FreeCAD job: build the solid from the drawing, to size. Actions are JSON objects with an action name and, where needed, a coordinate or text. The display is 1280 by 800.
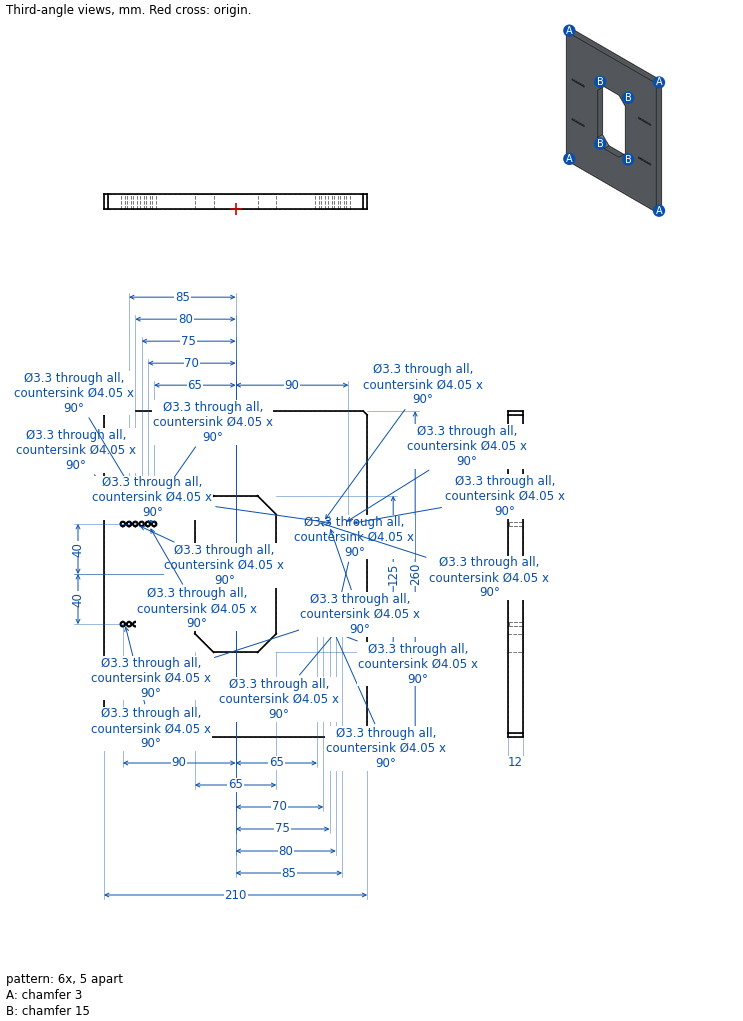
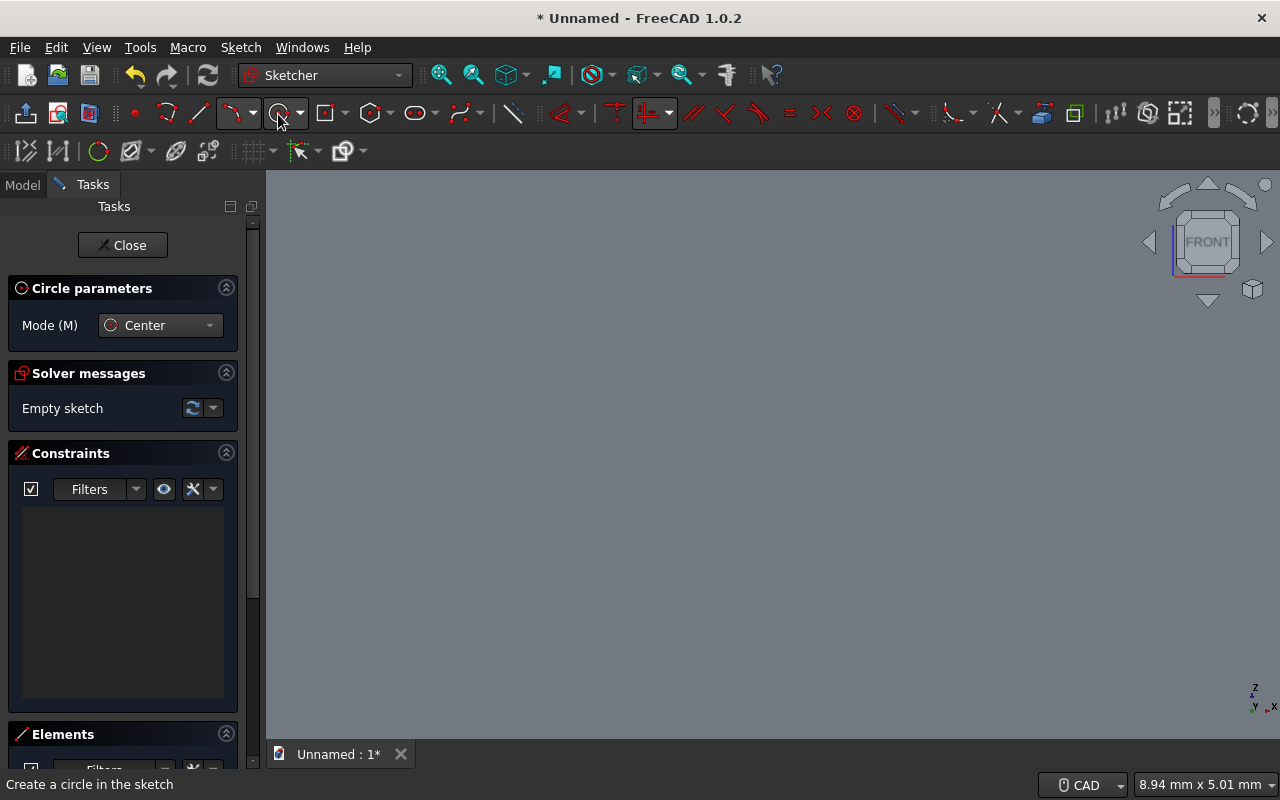
{"action": "left_click", "coordinate": [704, 453]}
{"action": "mouse_move", "coordinate": [836, 320]}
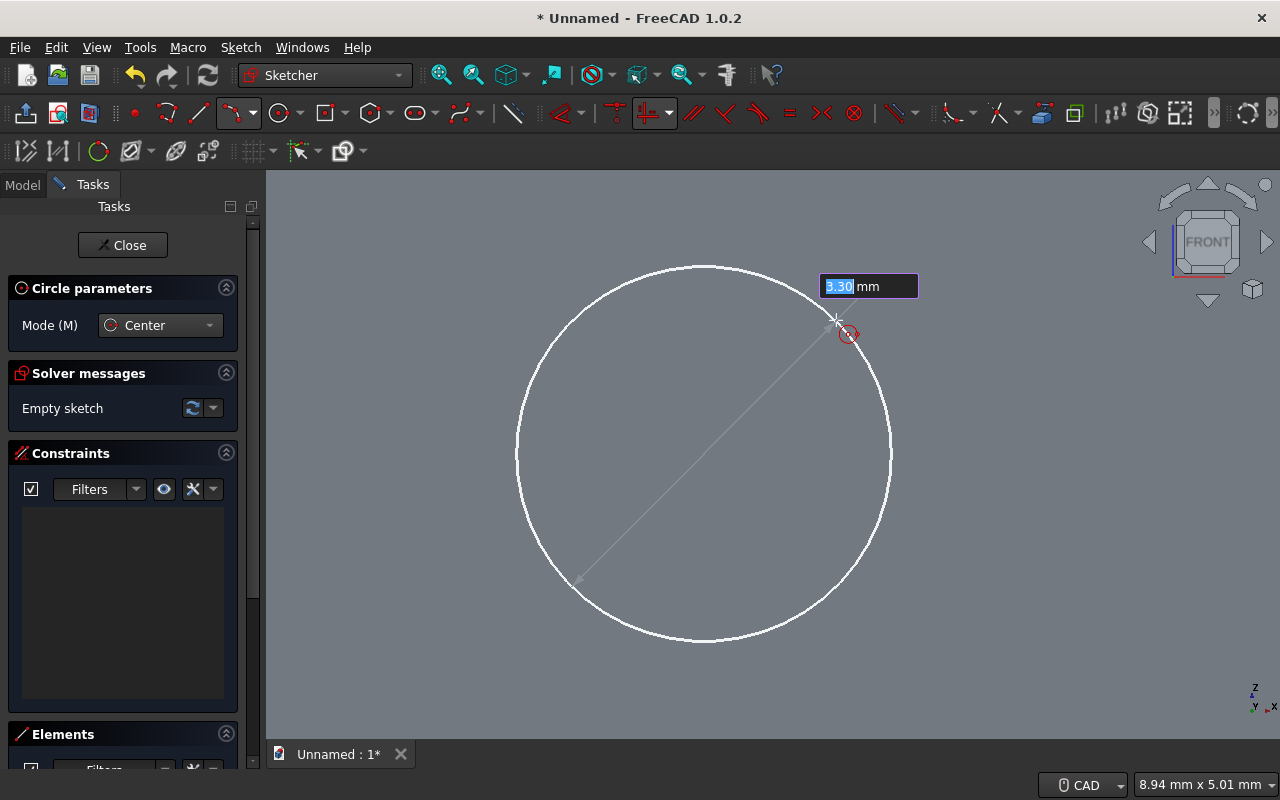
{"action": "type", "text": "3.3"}
{"action": "key", "text": "Return"}
{"action": "key", "text": "Escape"}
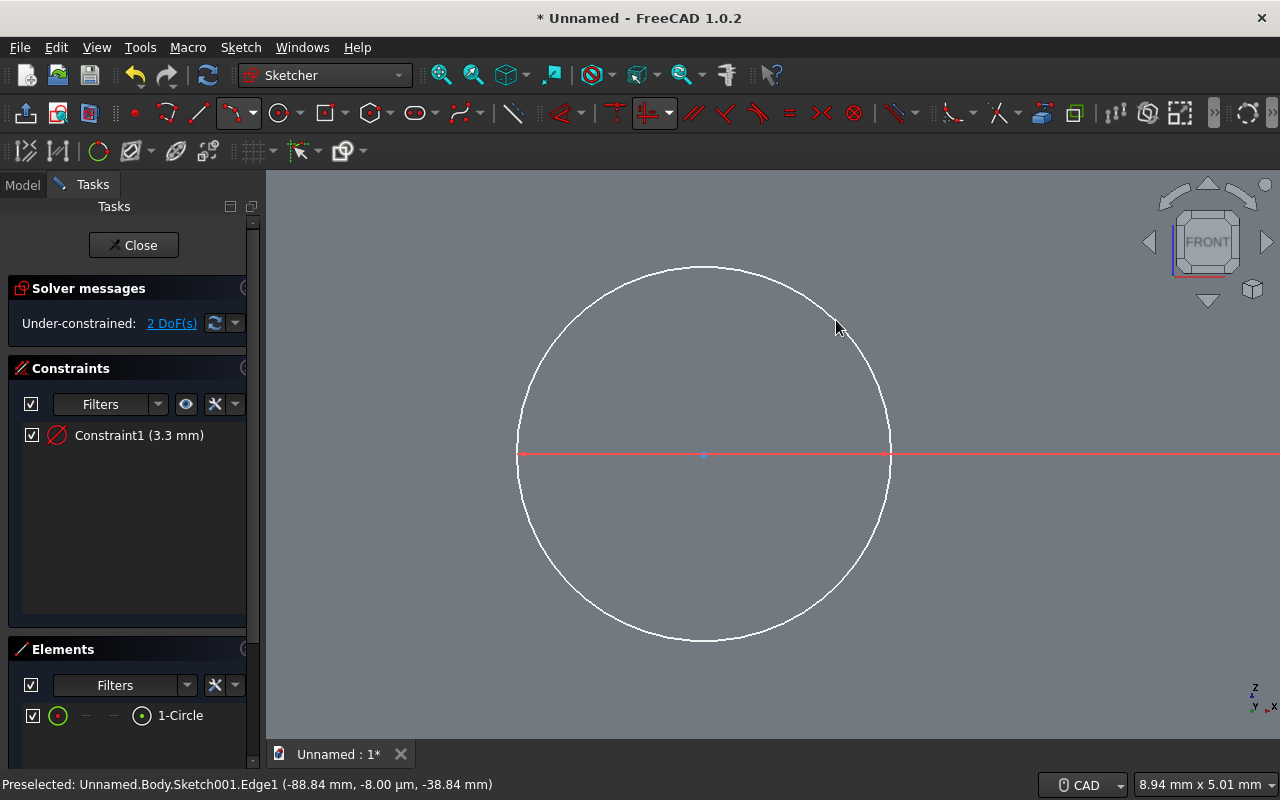
{"action": "left_click", "coordinate": [704, 454]}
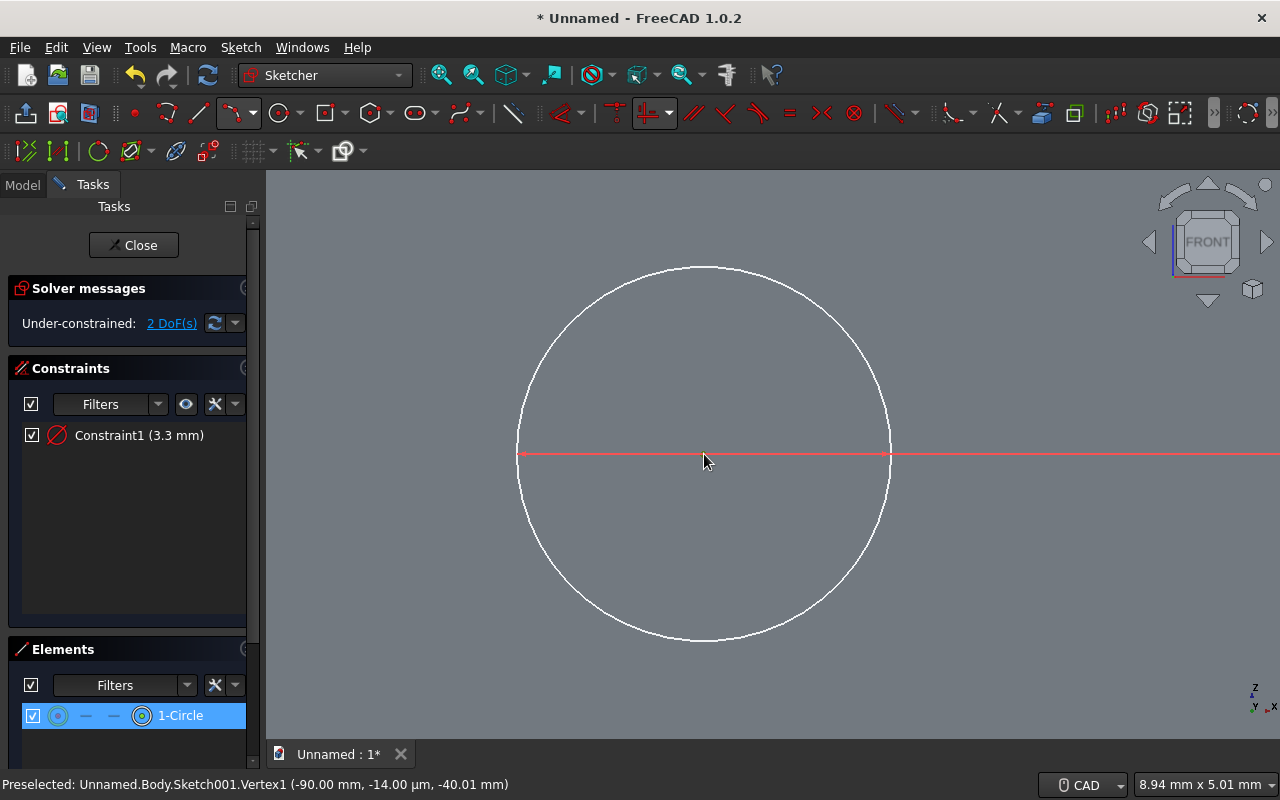
{"action": "key", "text": "l"}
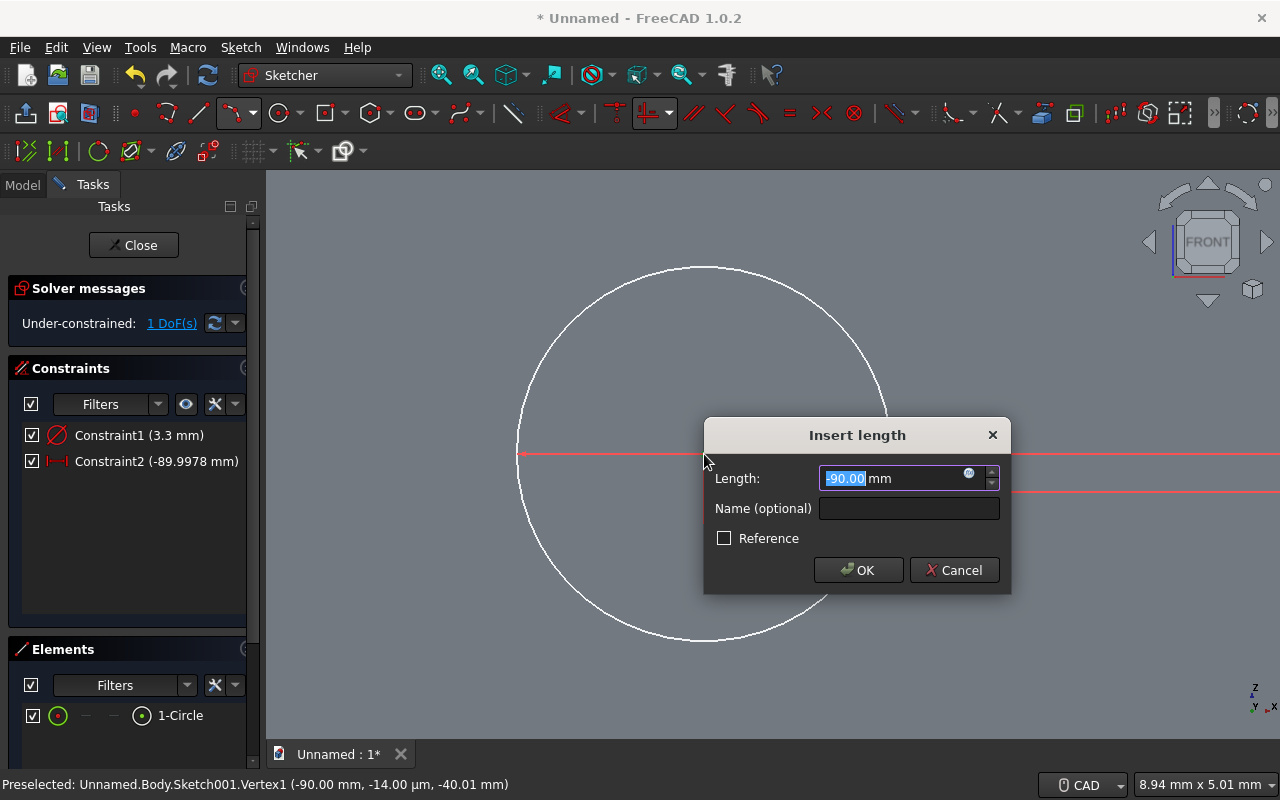
{"action": "type", "text": "-90"}
{"action": "key", "text": "Return"}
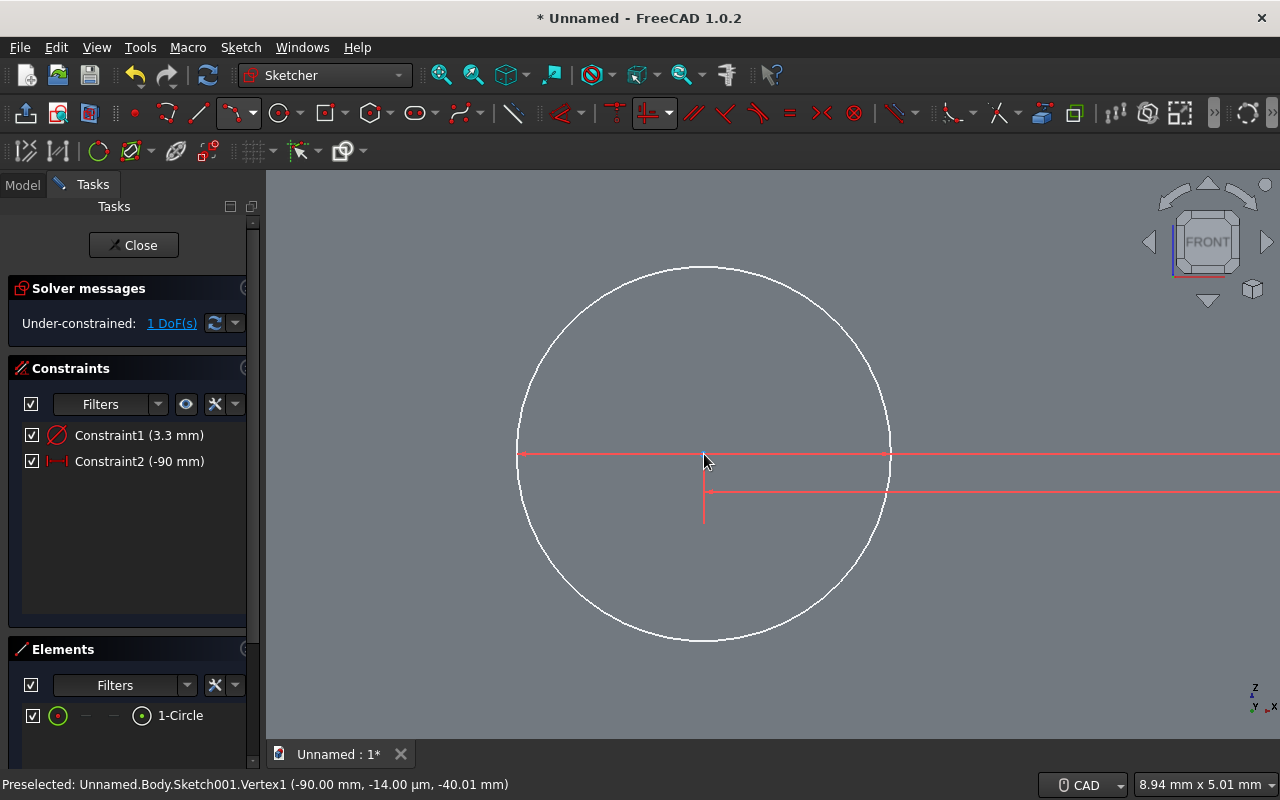
{"action": "left_click", "coordinate": [704, 454]}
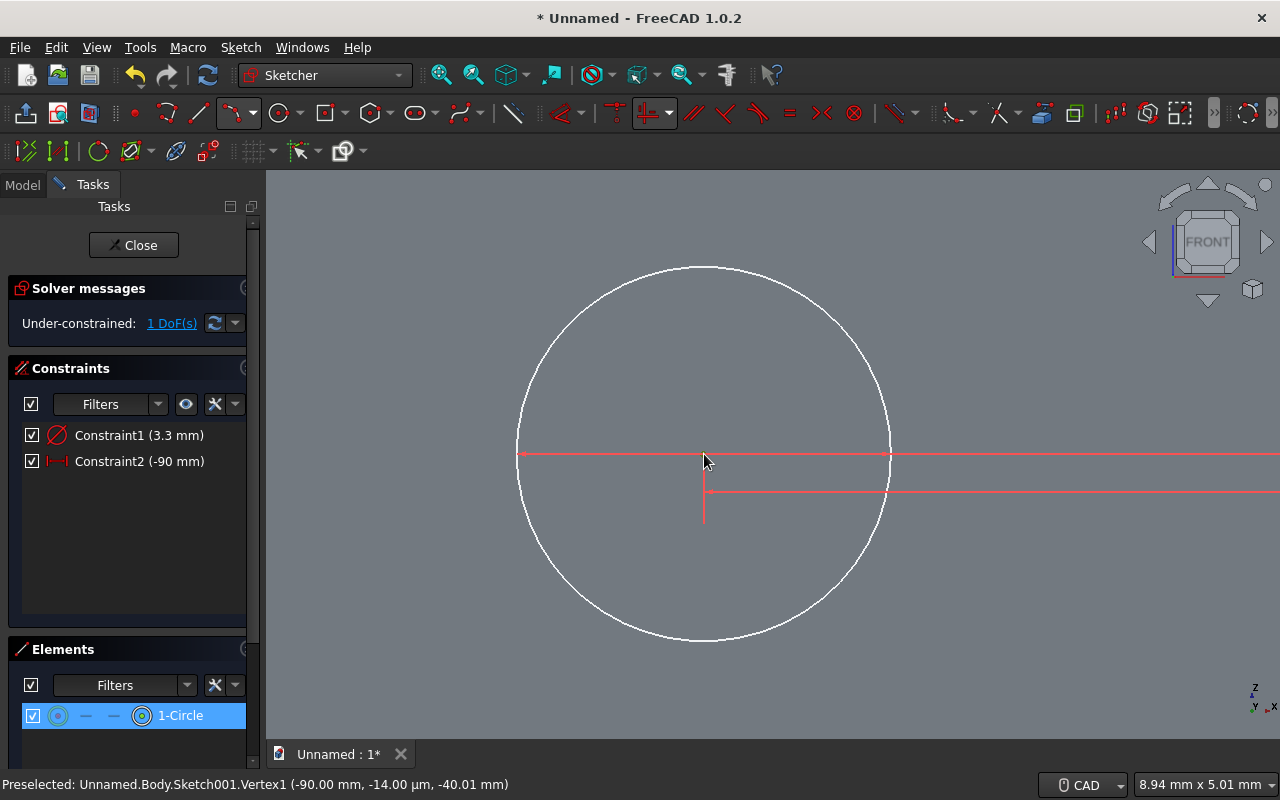
{"action": "left_click", "coordinate": [584, 114]}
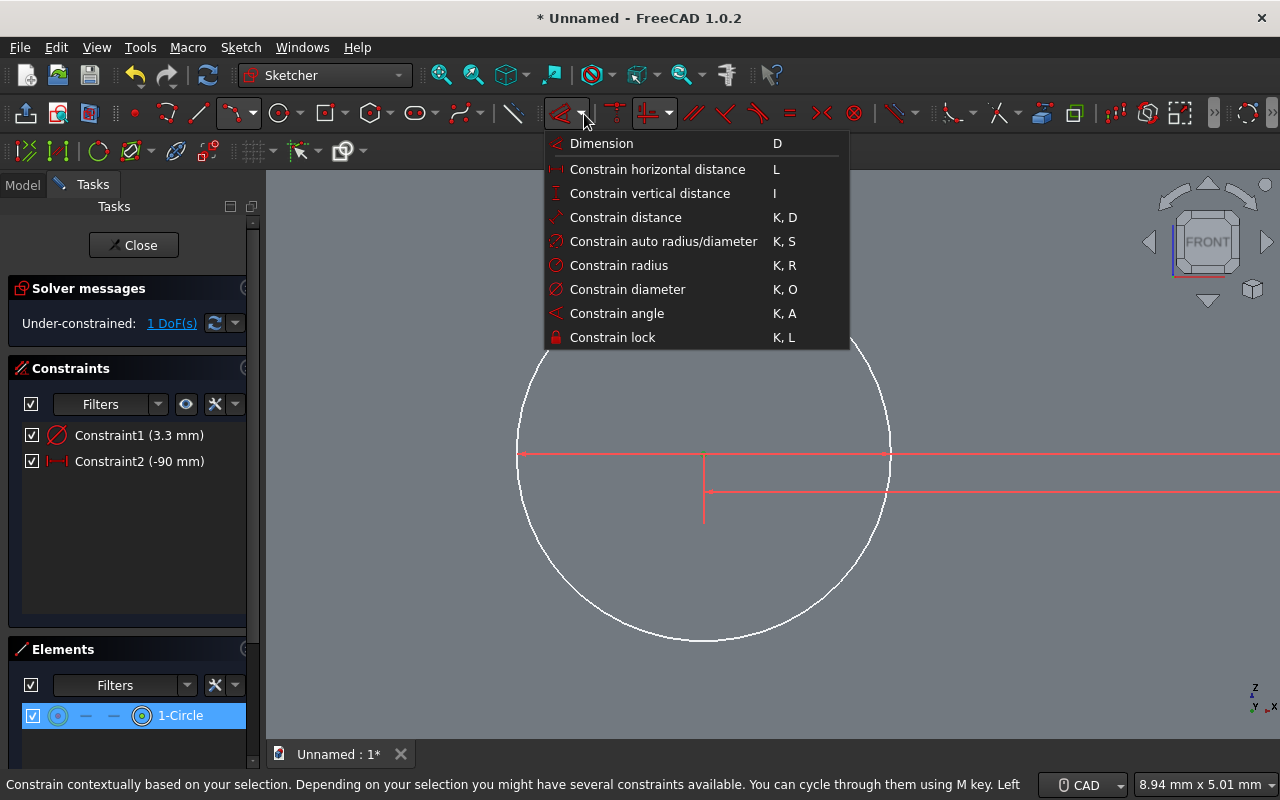
{"action": "left_click", "coordinate": [697, 193]}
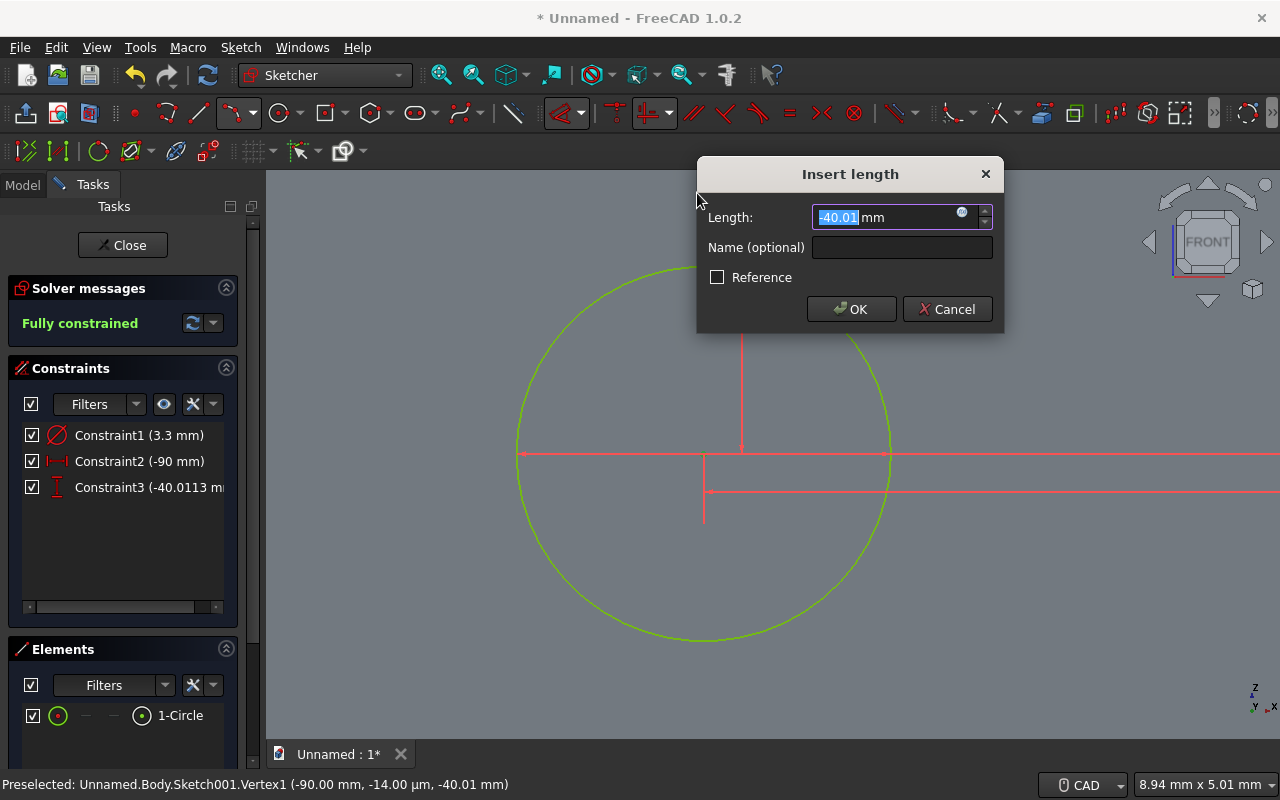
{"action": "type", "text": "-40"}
{"action": "key", "text": "Return"}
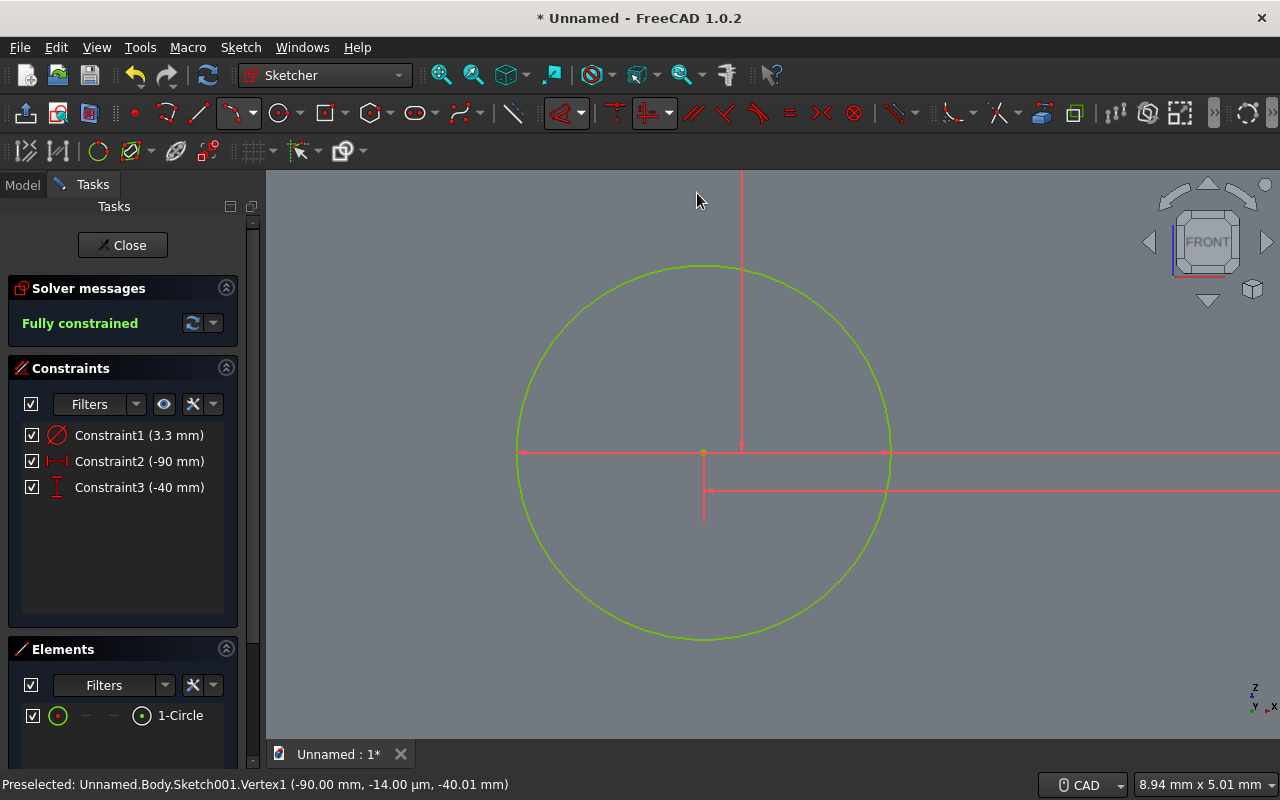
{"action": "left_click", "coordinate": [123, 245]}